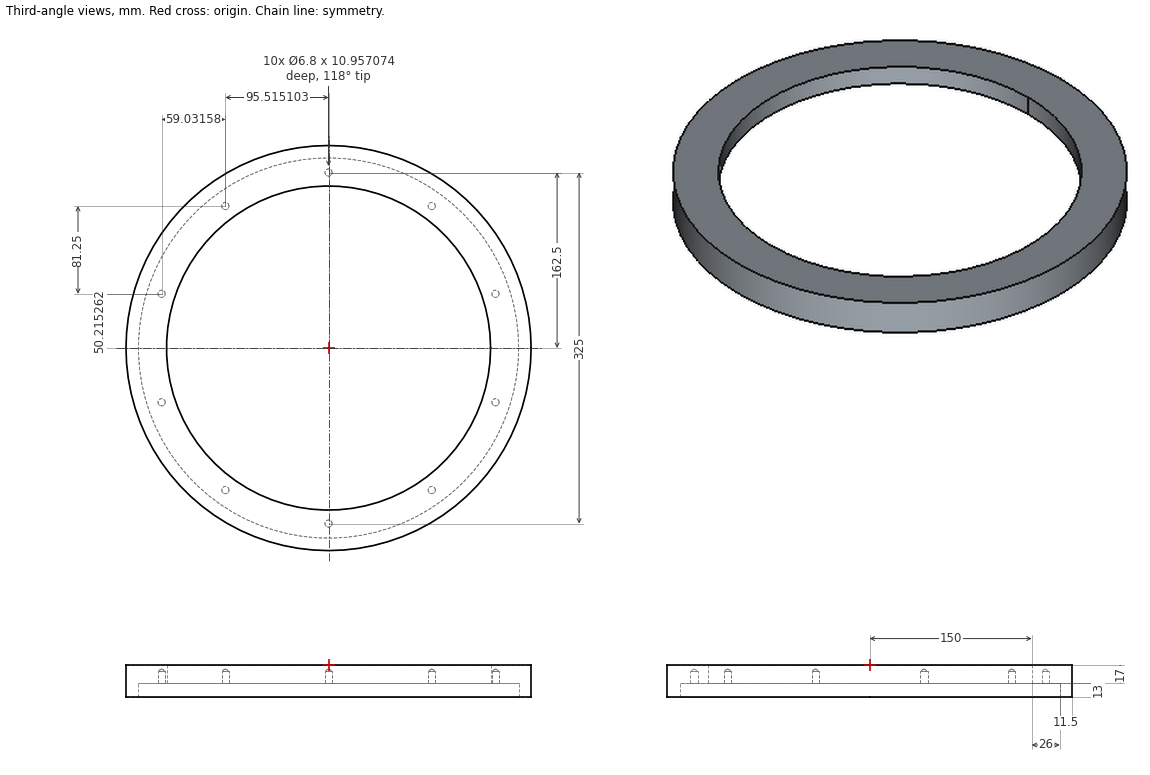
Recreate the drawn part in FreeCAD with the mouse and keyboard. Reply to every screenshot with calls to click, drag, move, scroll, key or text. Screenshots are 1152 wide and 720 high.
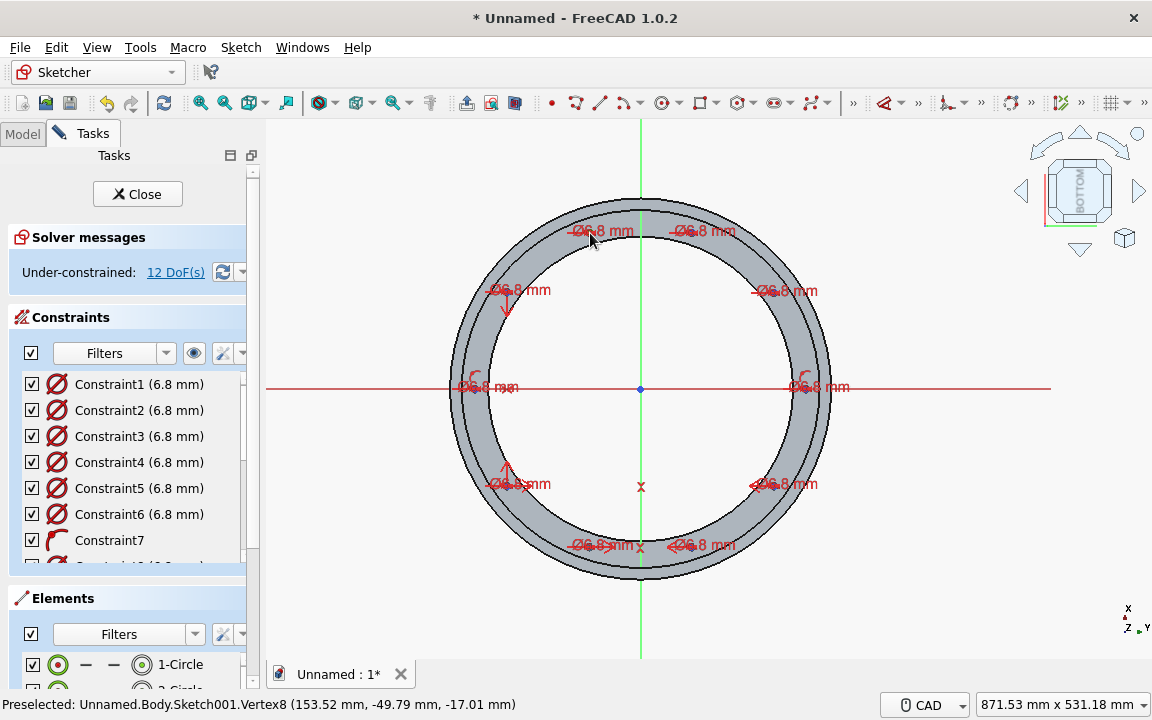
click(344, 389)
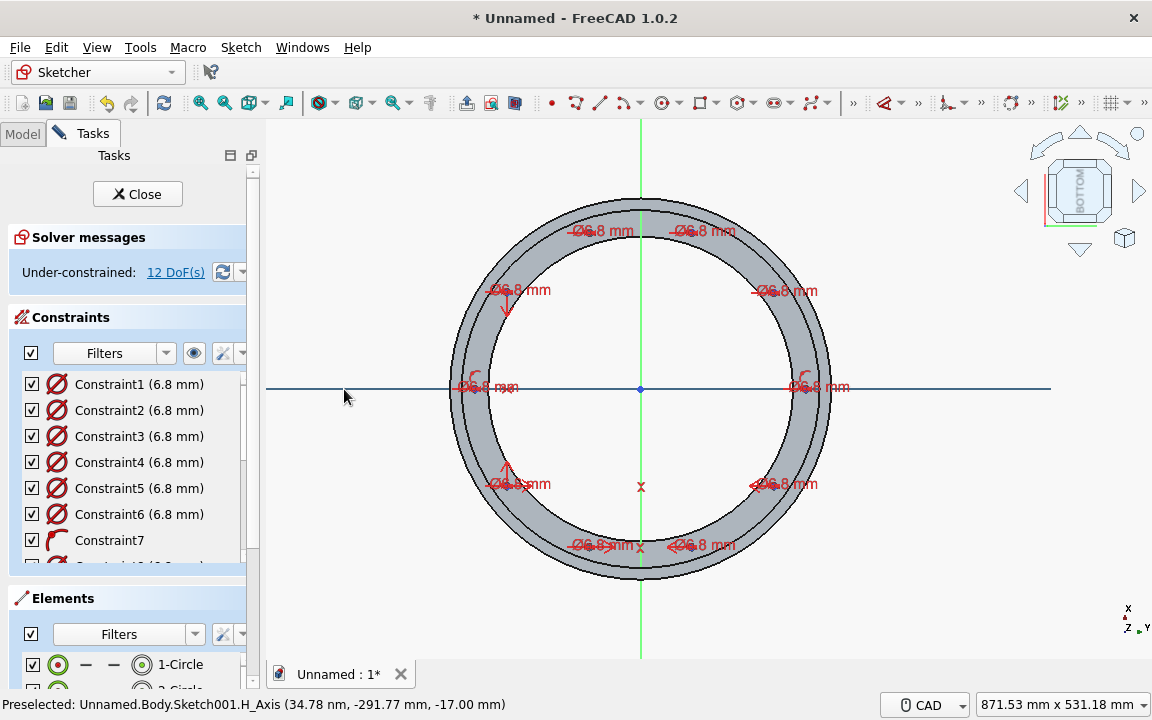
key(s)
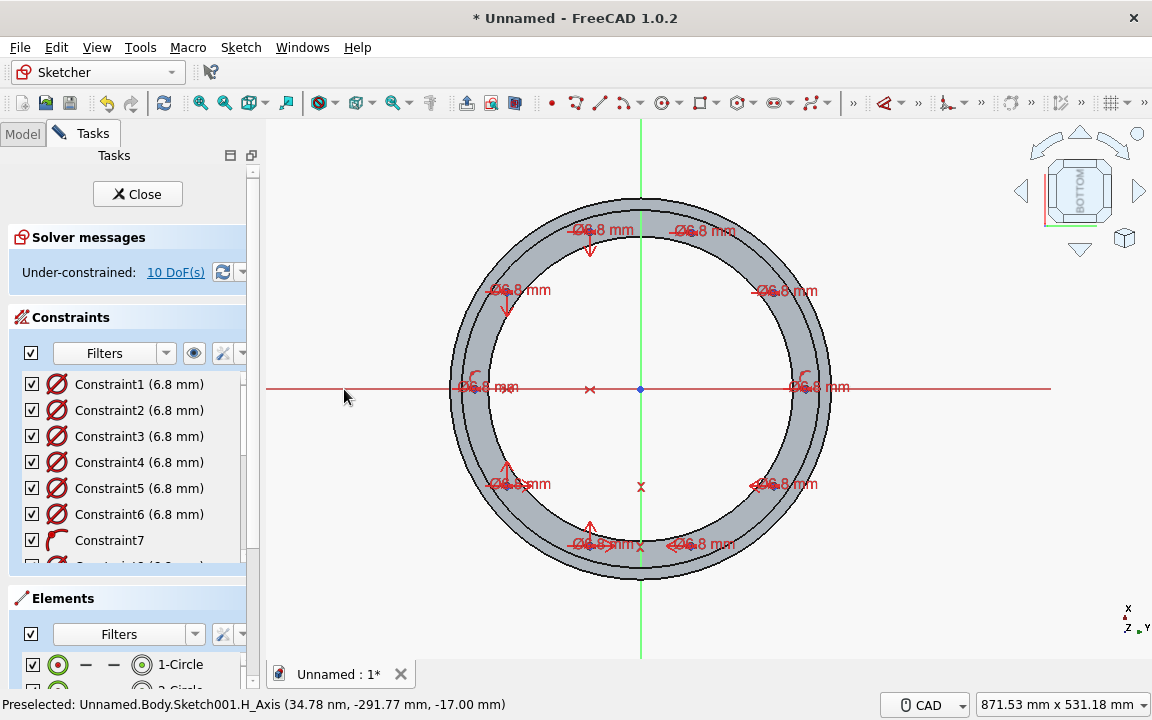
click(691, 546)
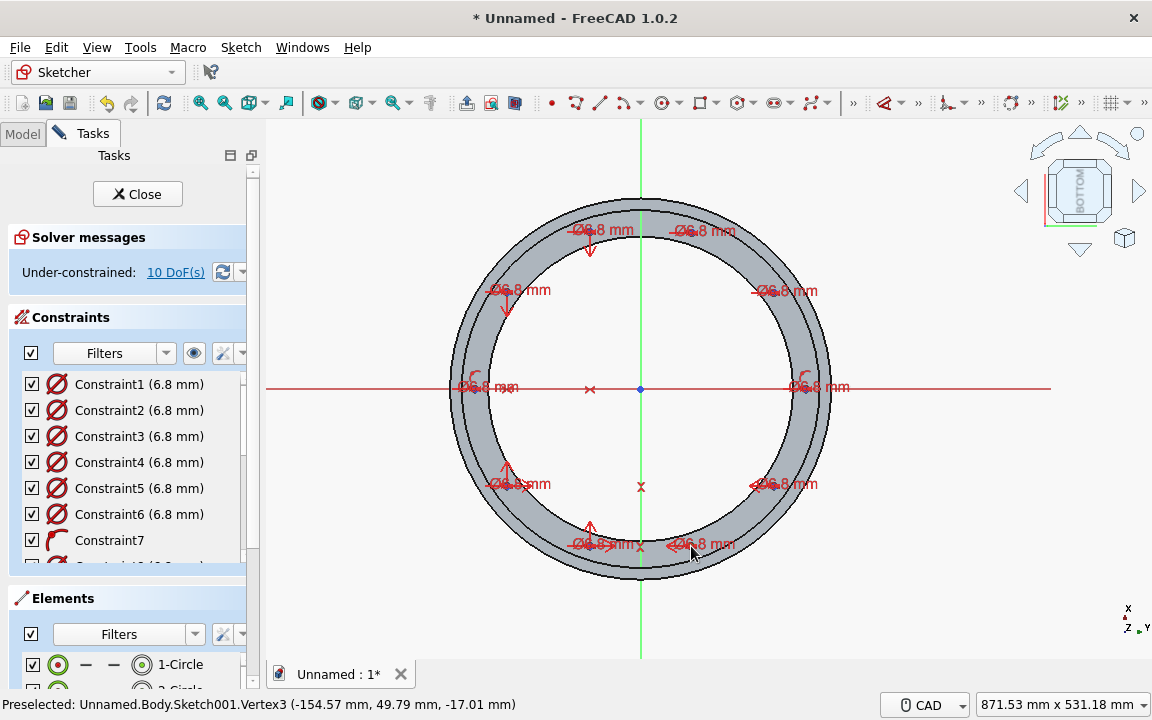
click(692, 233)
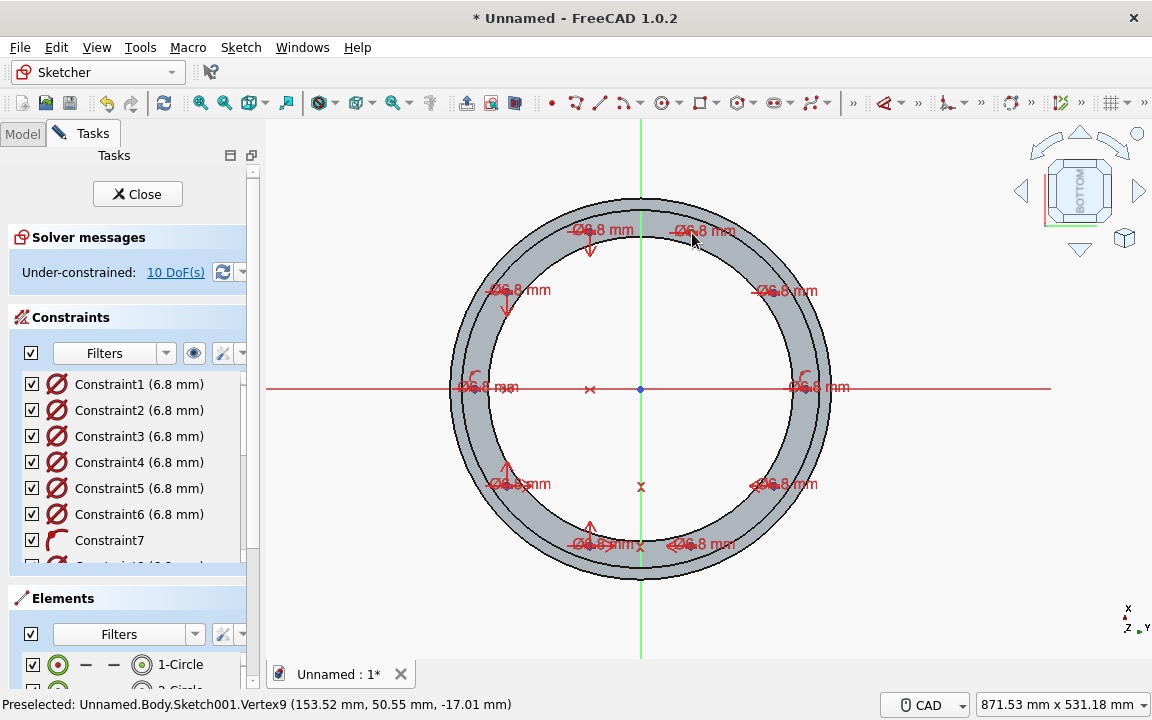
click(344, 389)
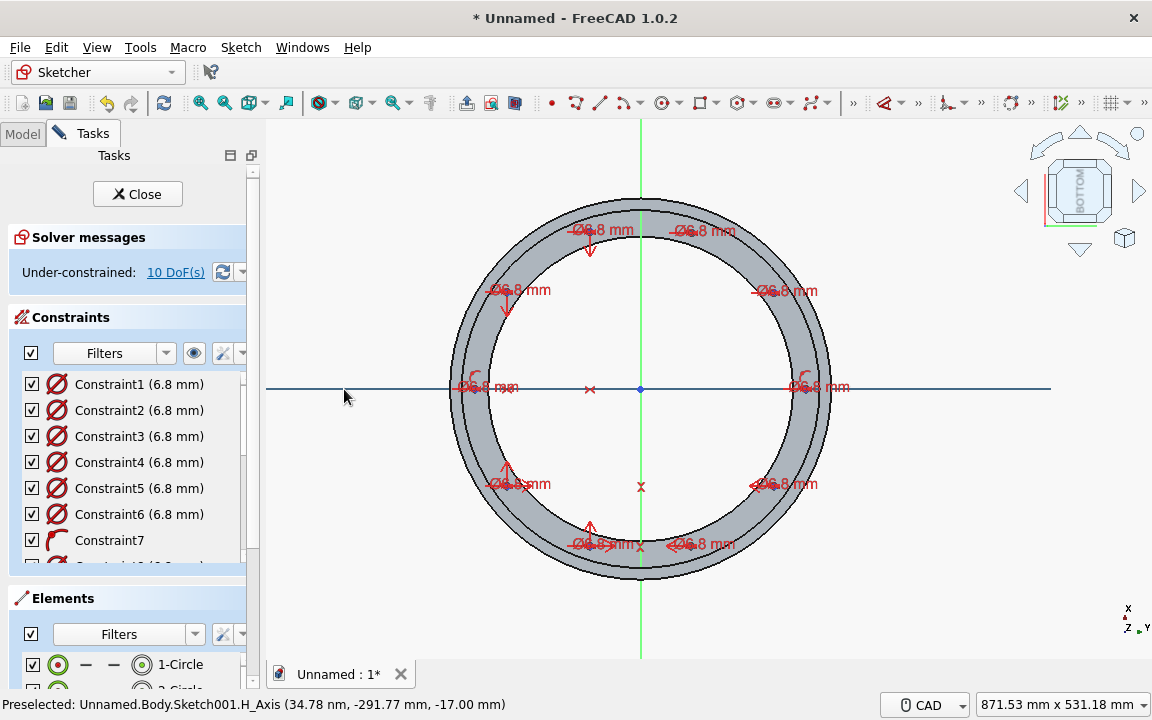
key(s)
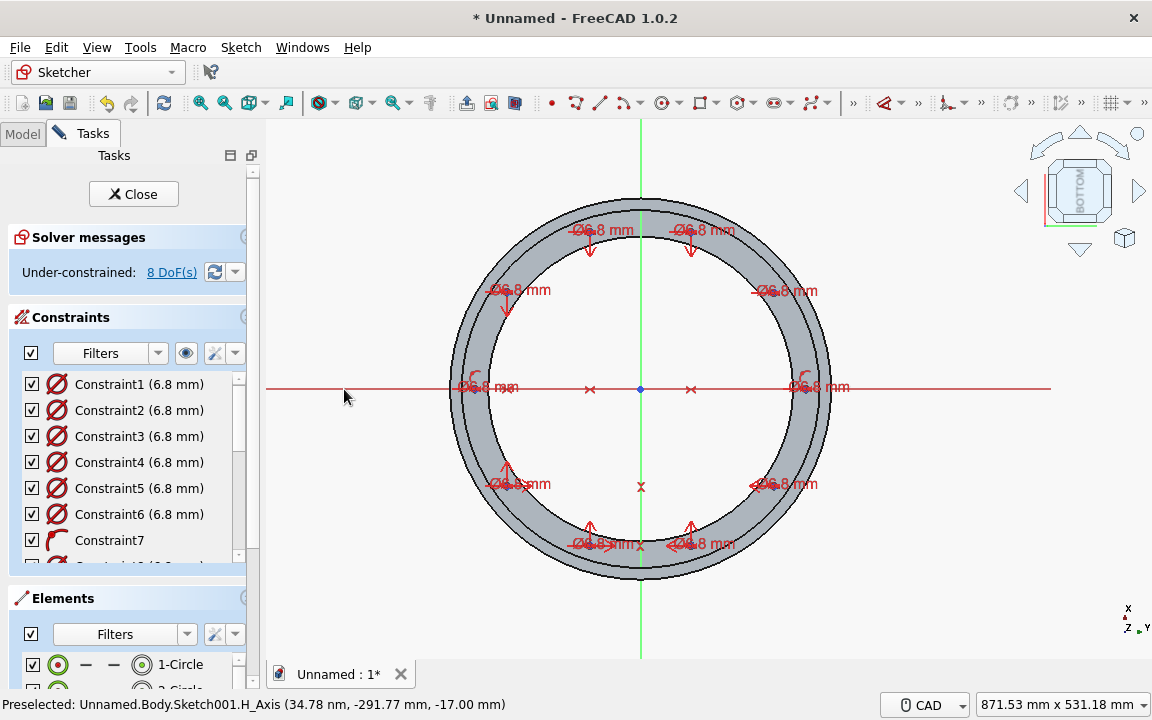
click(774, 486)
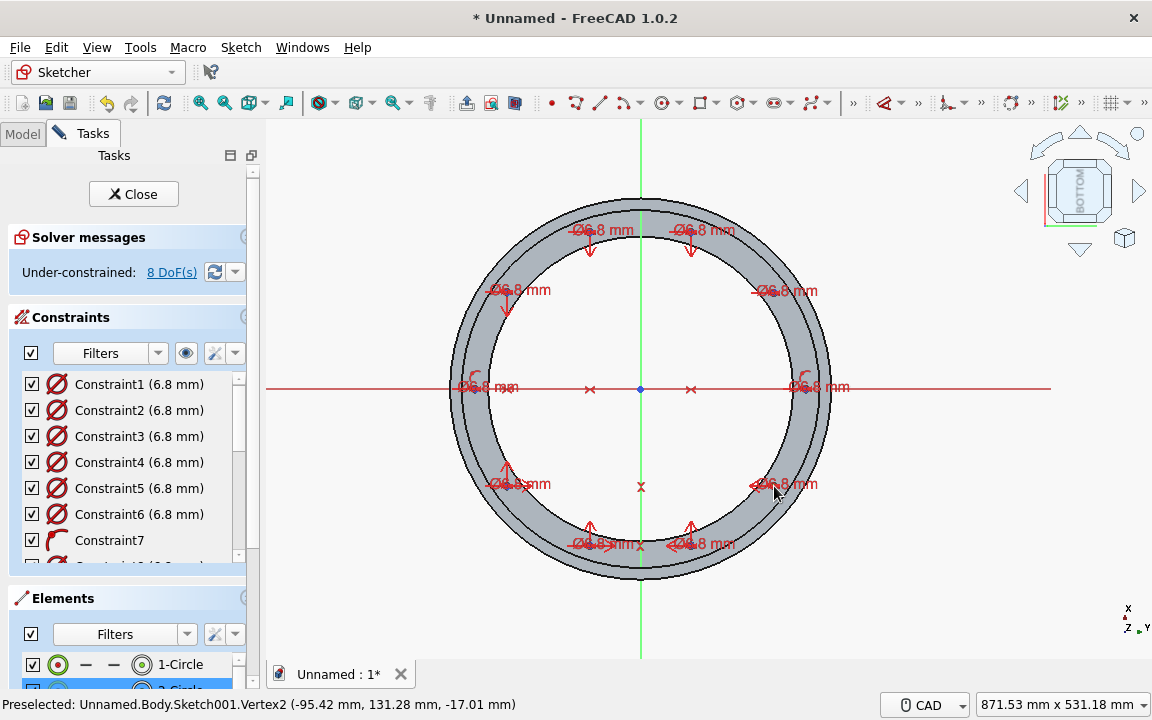
click(774, 293)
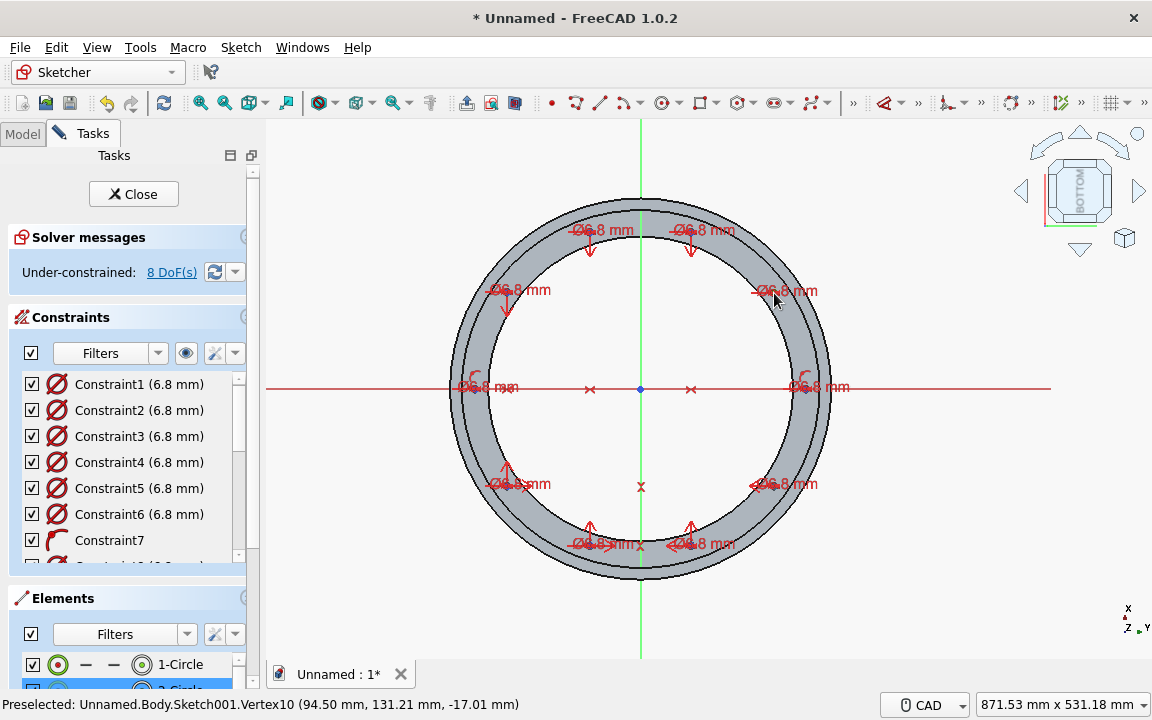
click(344, 389)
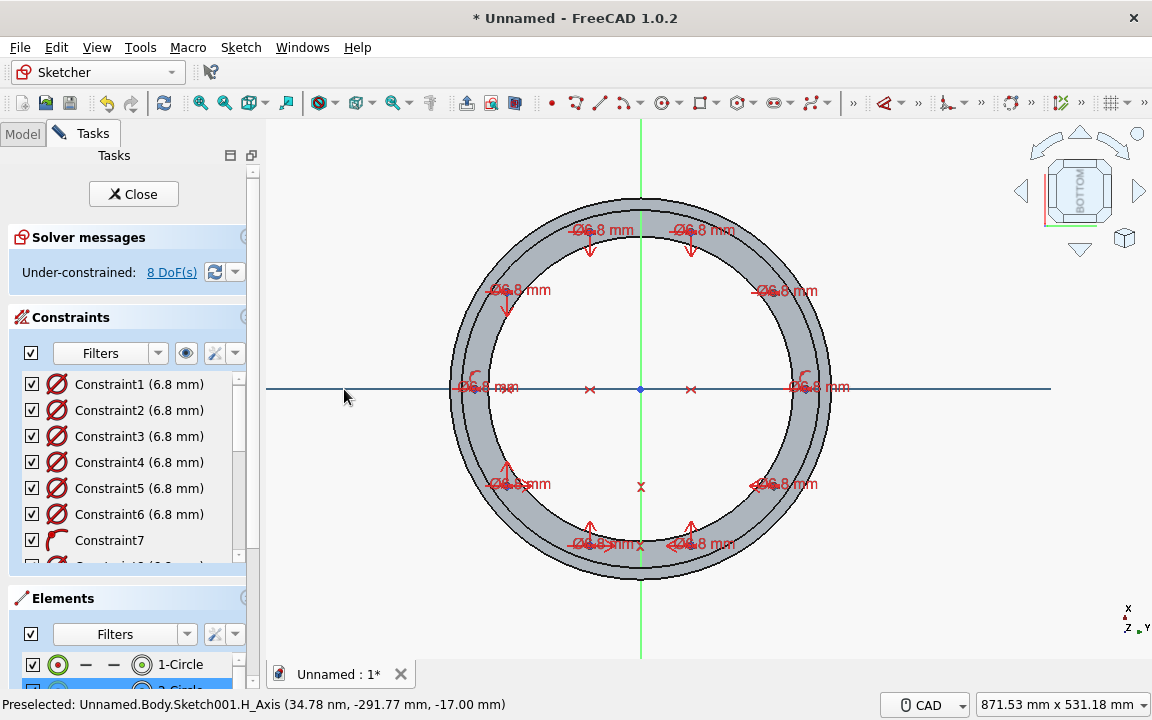
key(s)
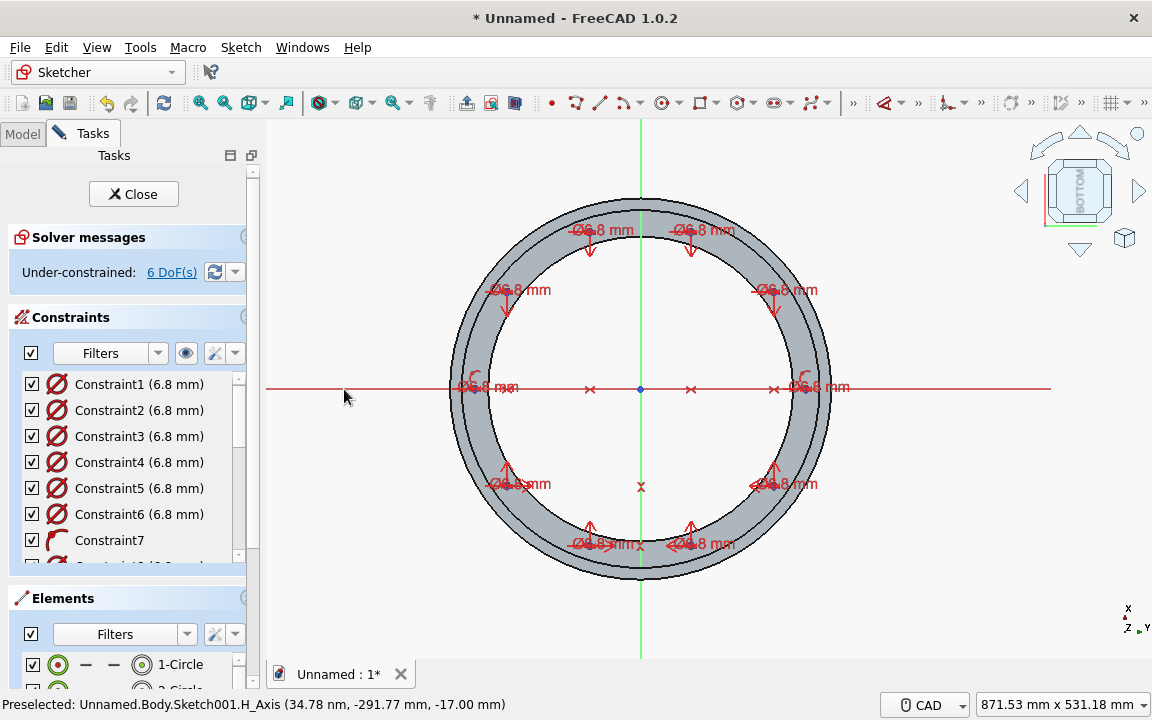
click(806, 389)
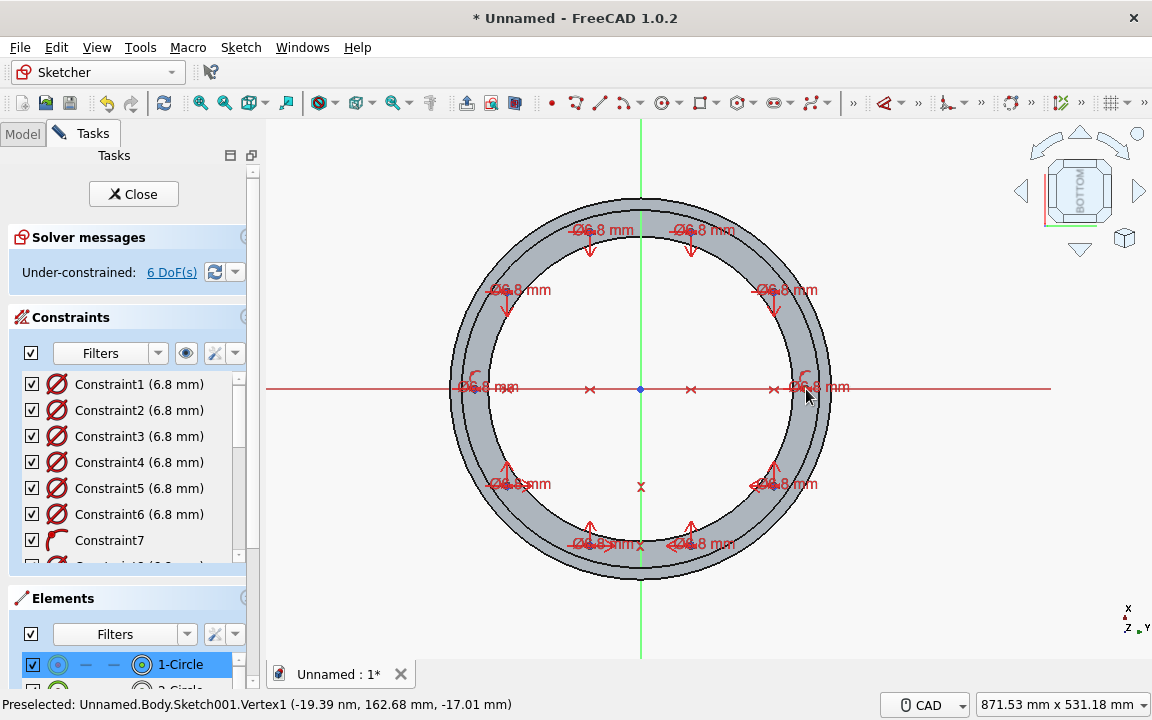
click(475, 389)